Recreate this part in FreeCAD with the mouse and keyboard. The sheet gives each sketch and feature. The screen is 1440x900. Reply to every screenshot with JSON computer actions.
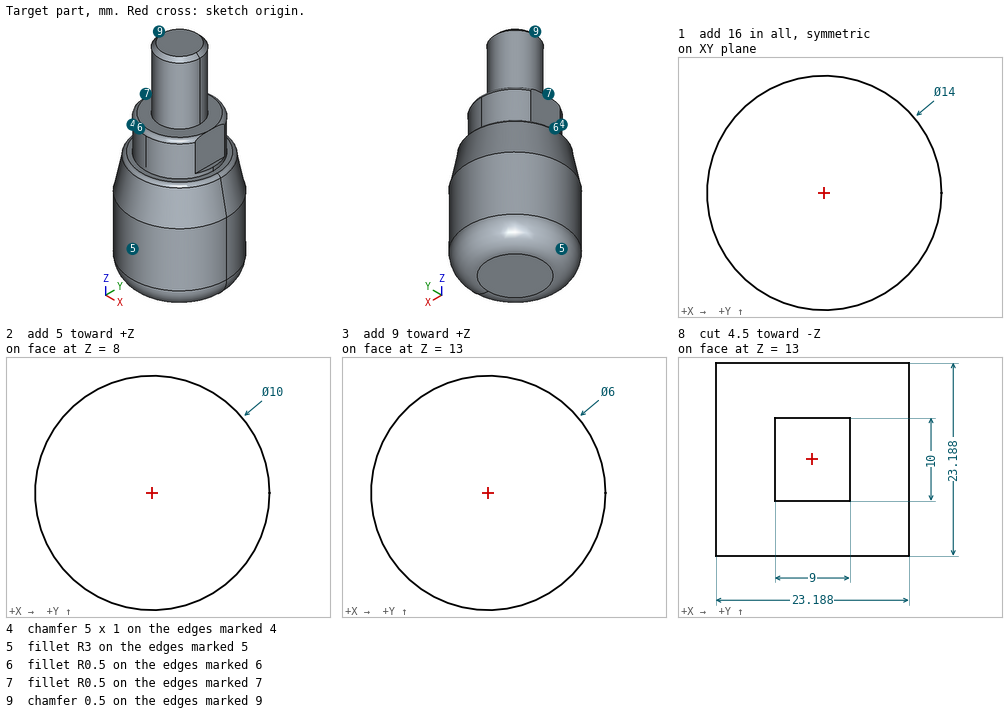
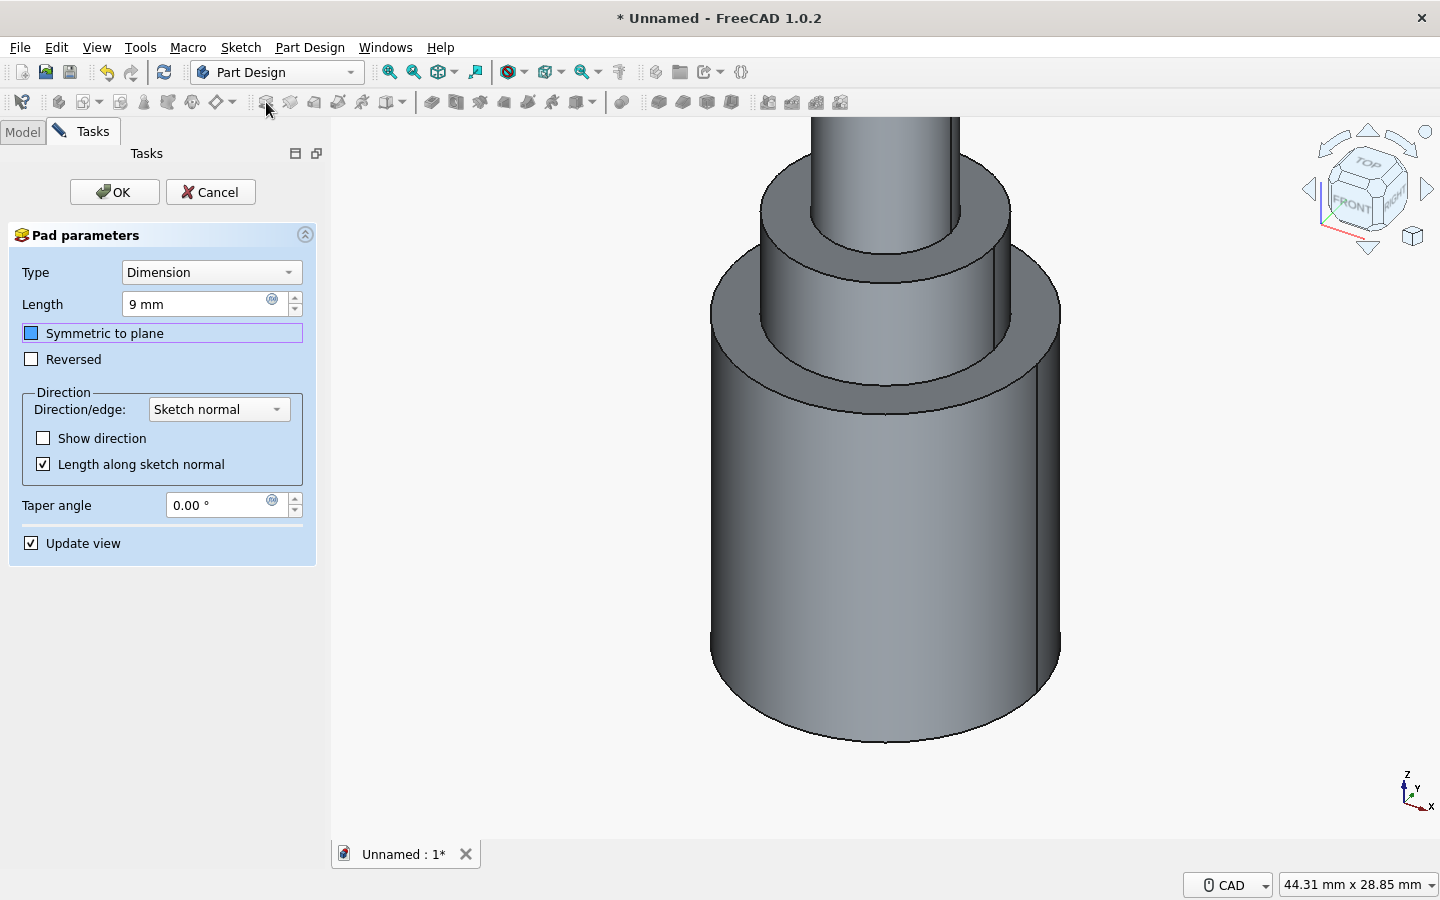
{"action": "left_click", "coordinate": [115, 192]}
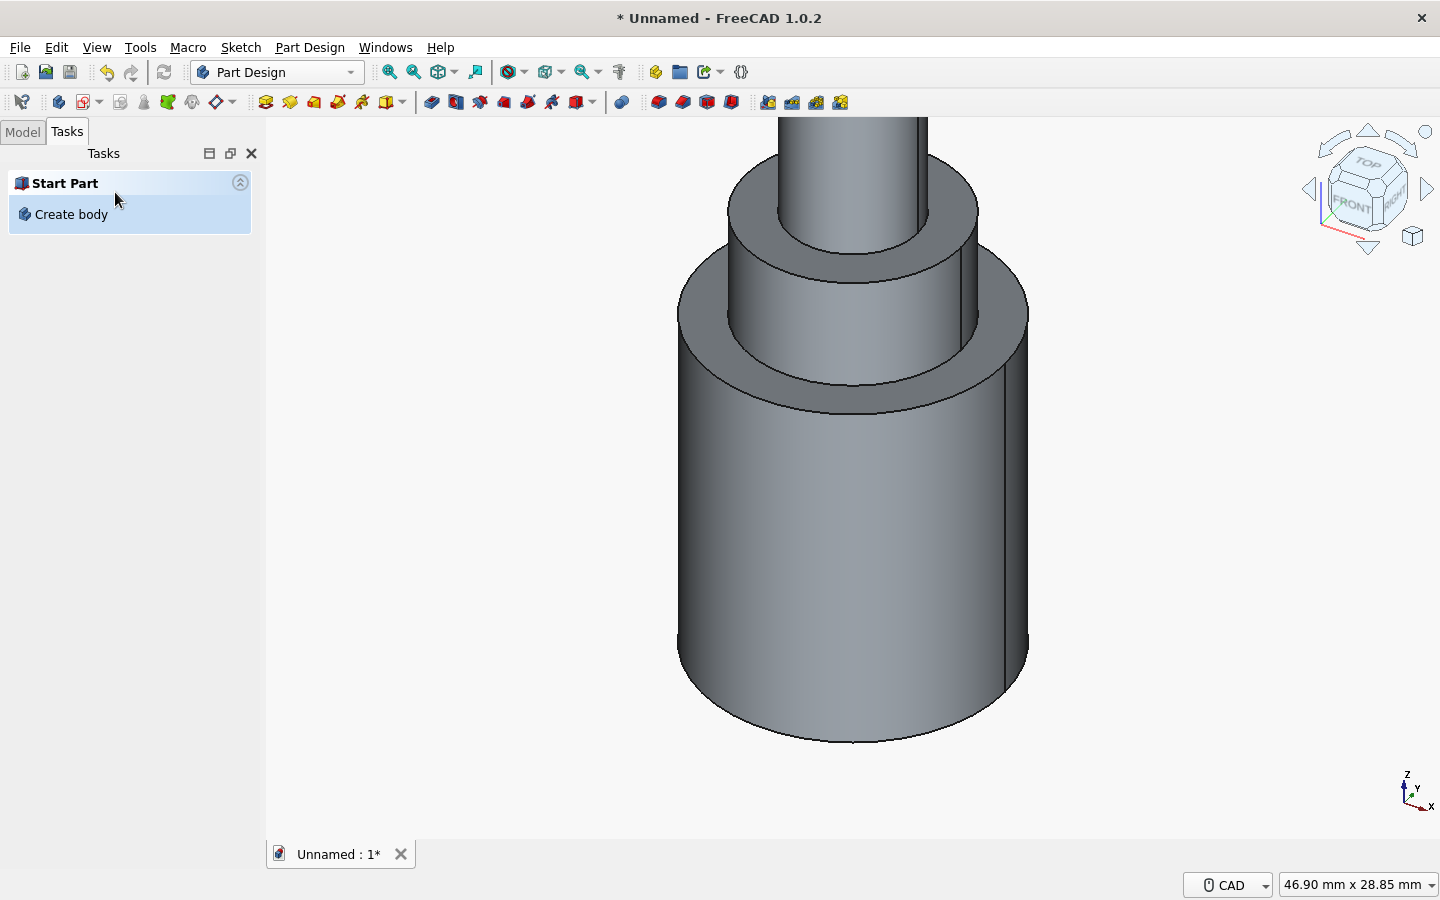
{"action": "key", "text": "v f"}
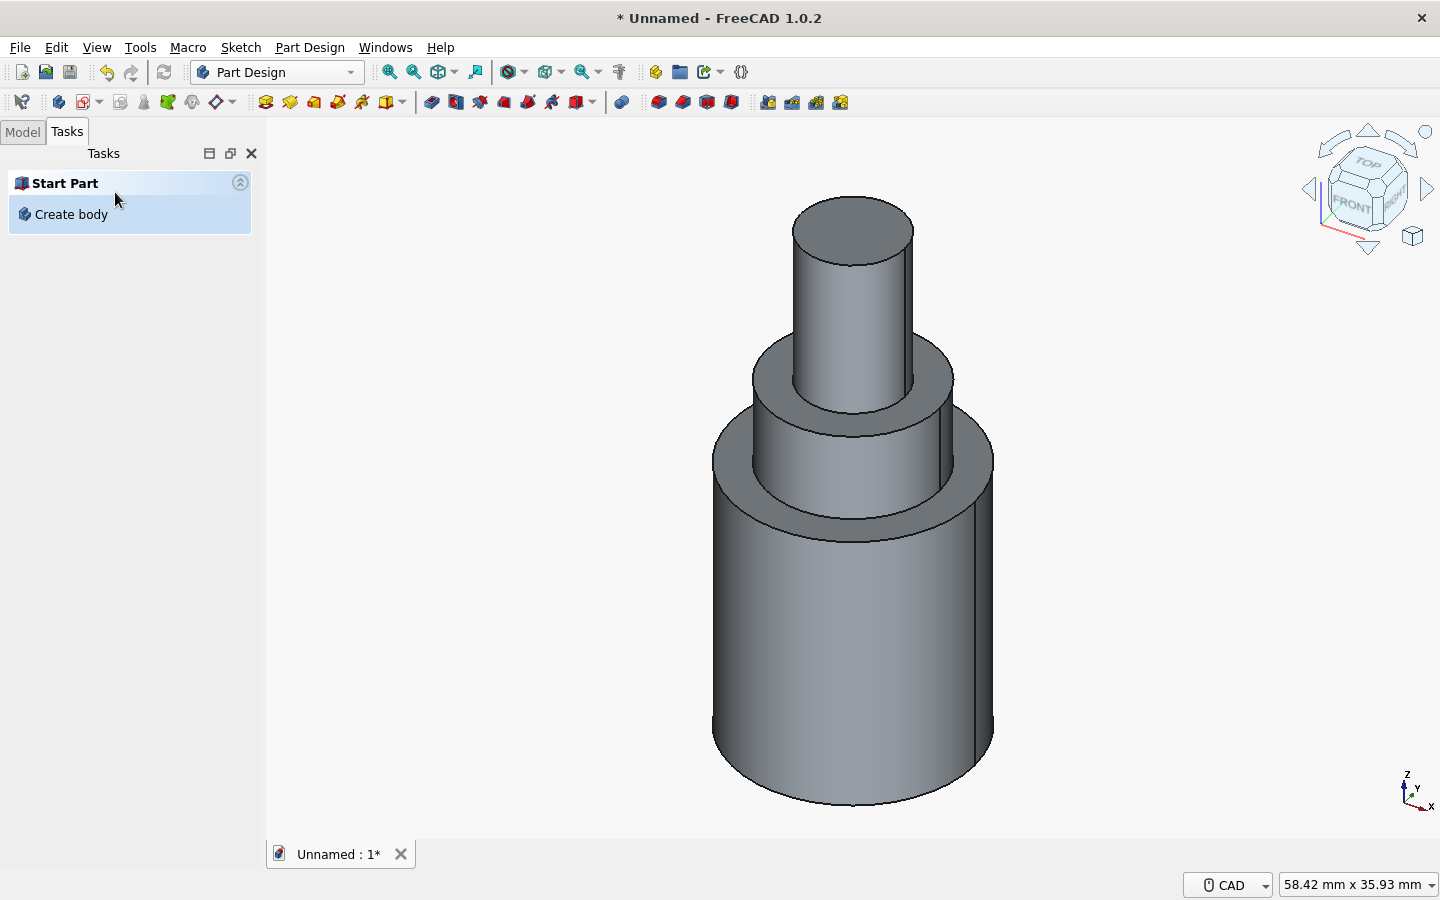
{"action": "left_click", "coordinate": [713, 469]}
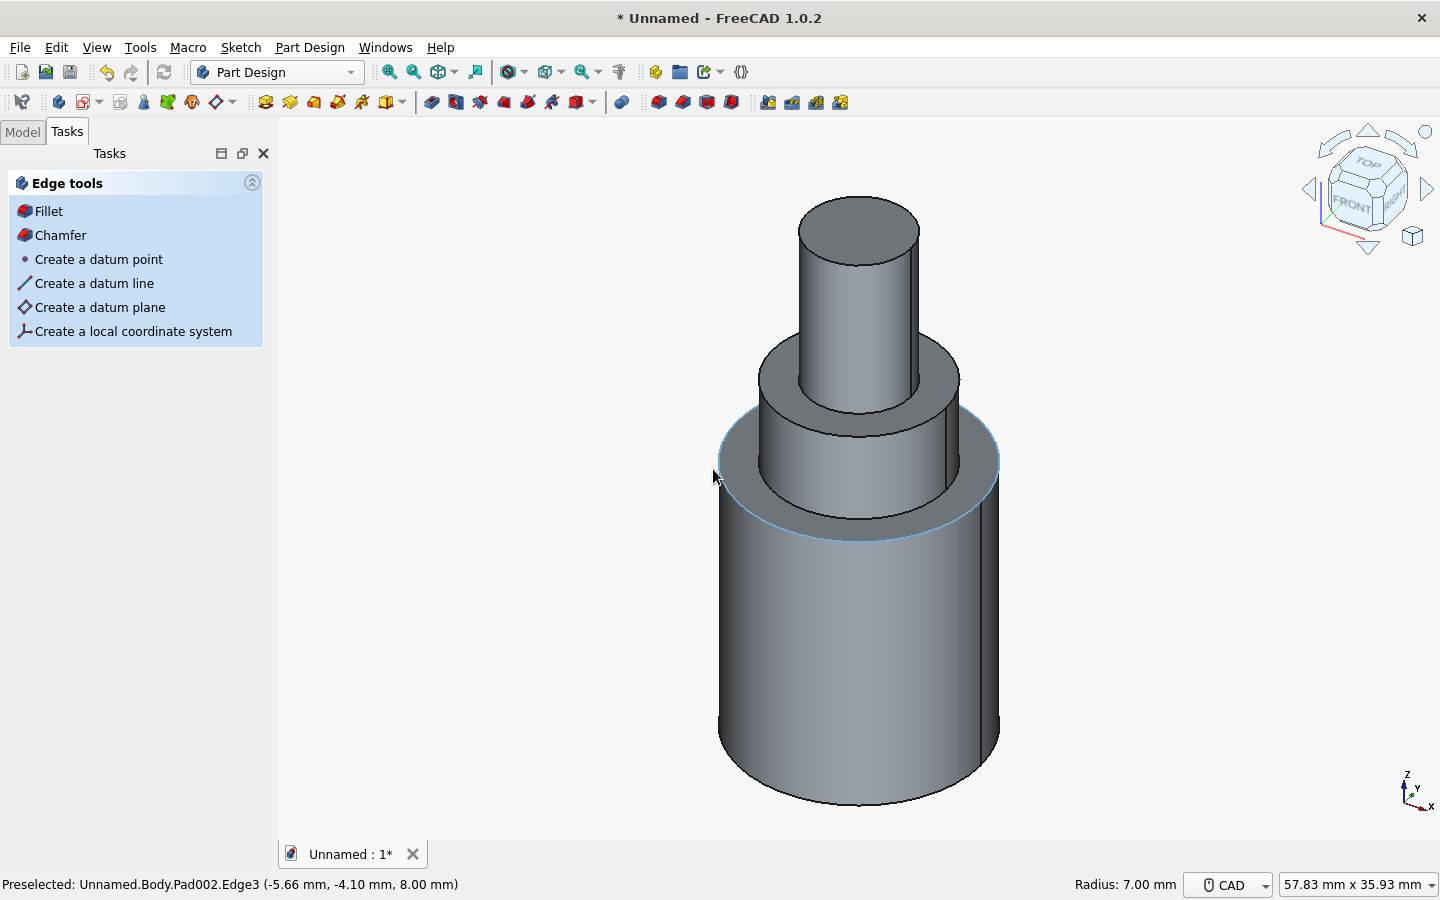
{"action": "left_click", "coordinate": [684, 102]}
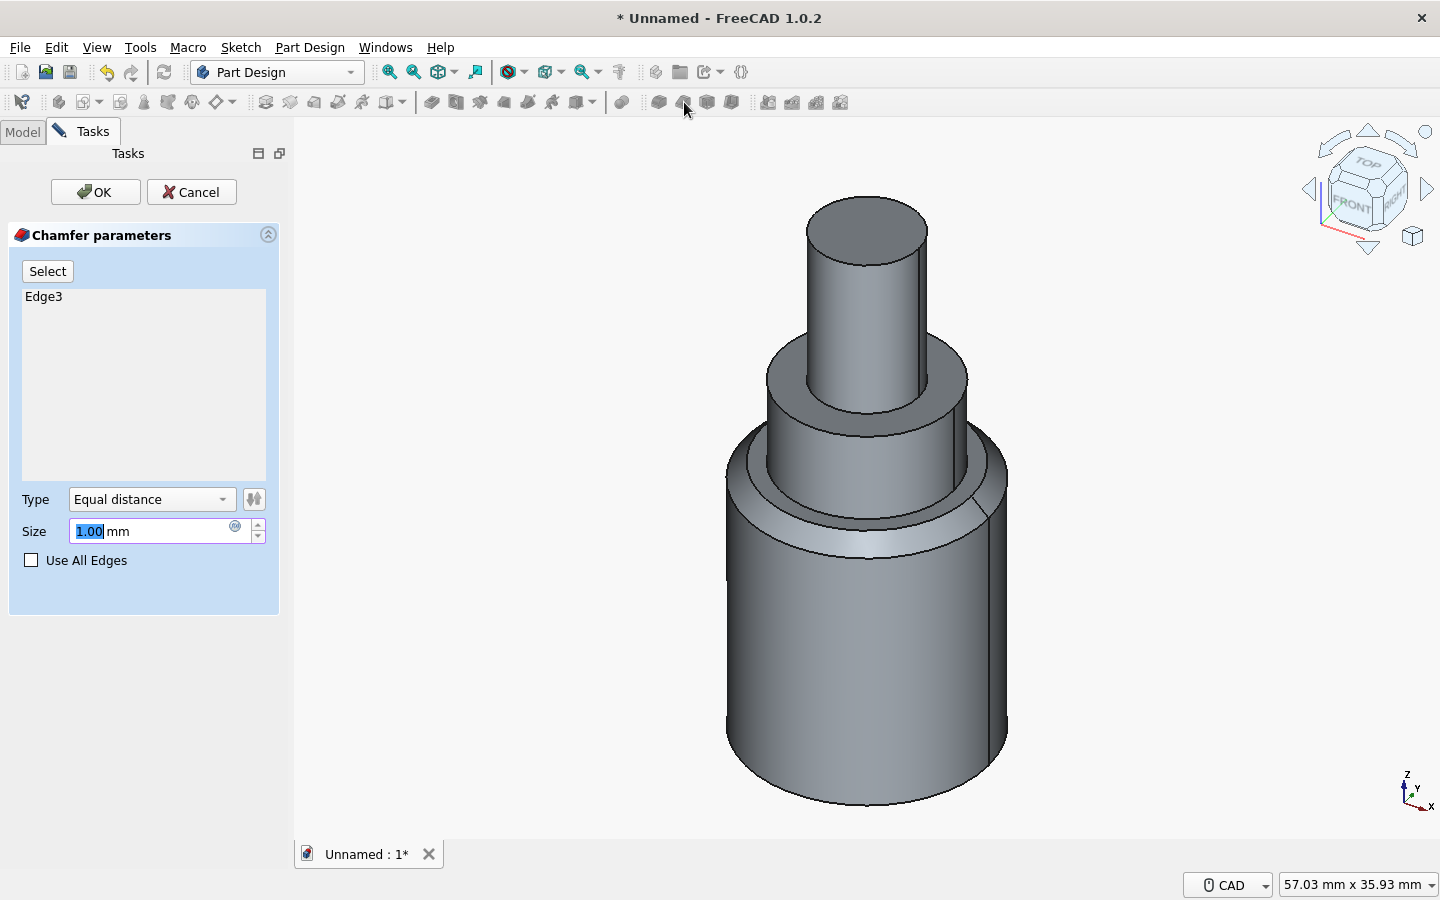
{"action": "type", "text": "5"}
{"action": "key", "text": "Tab"}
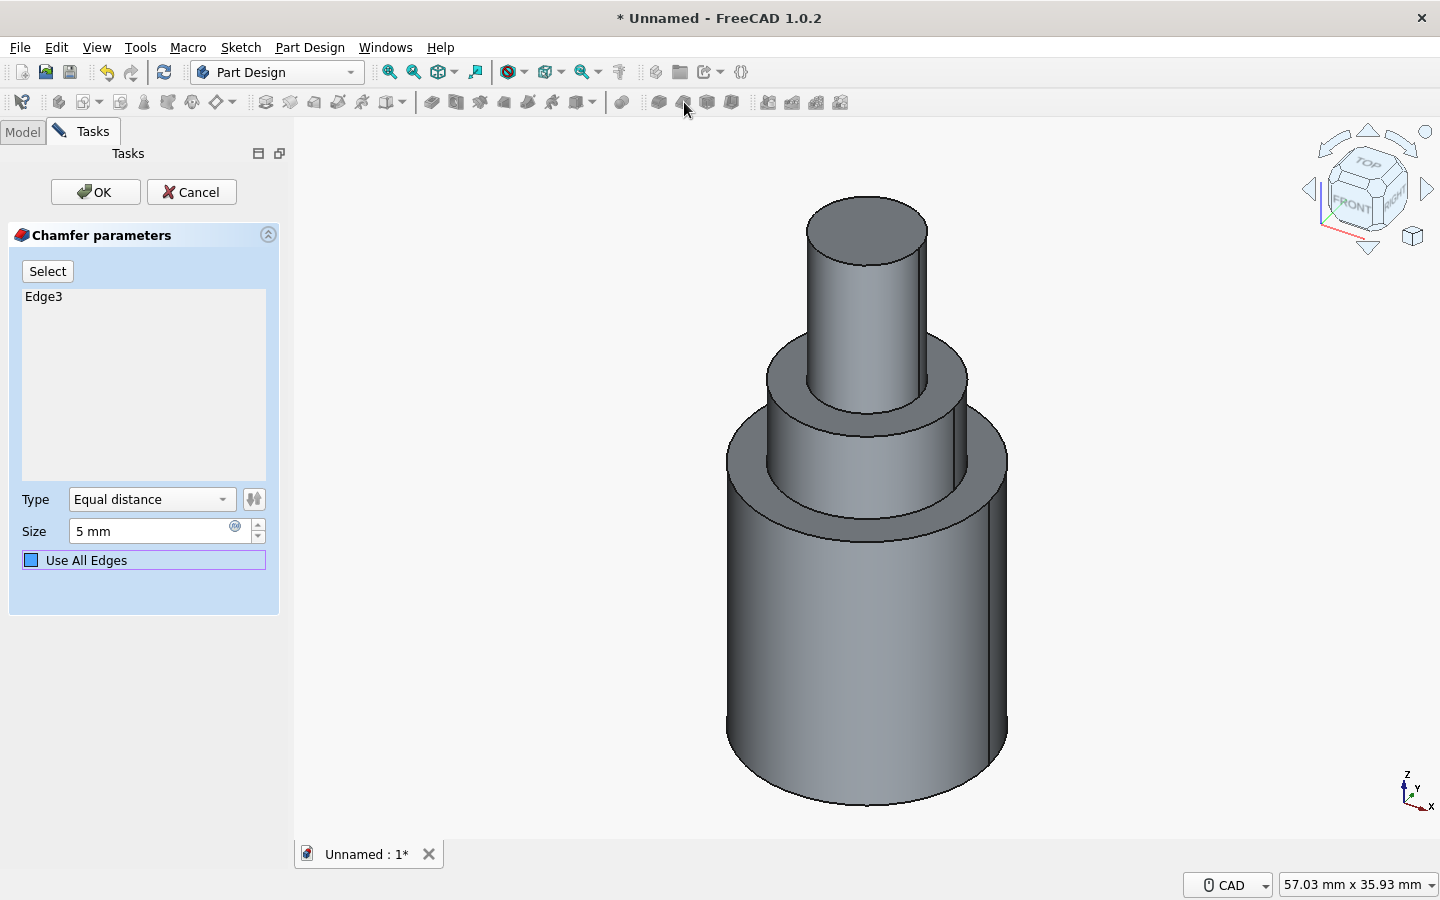
{"action": "left_click", "coordinate": [153, 500]}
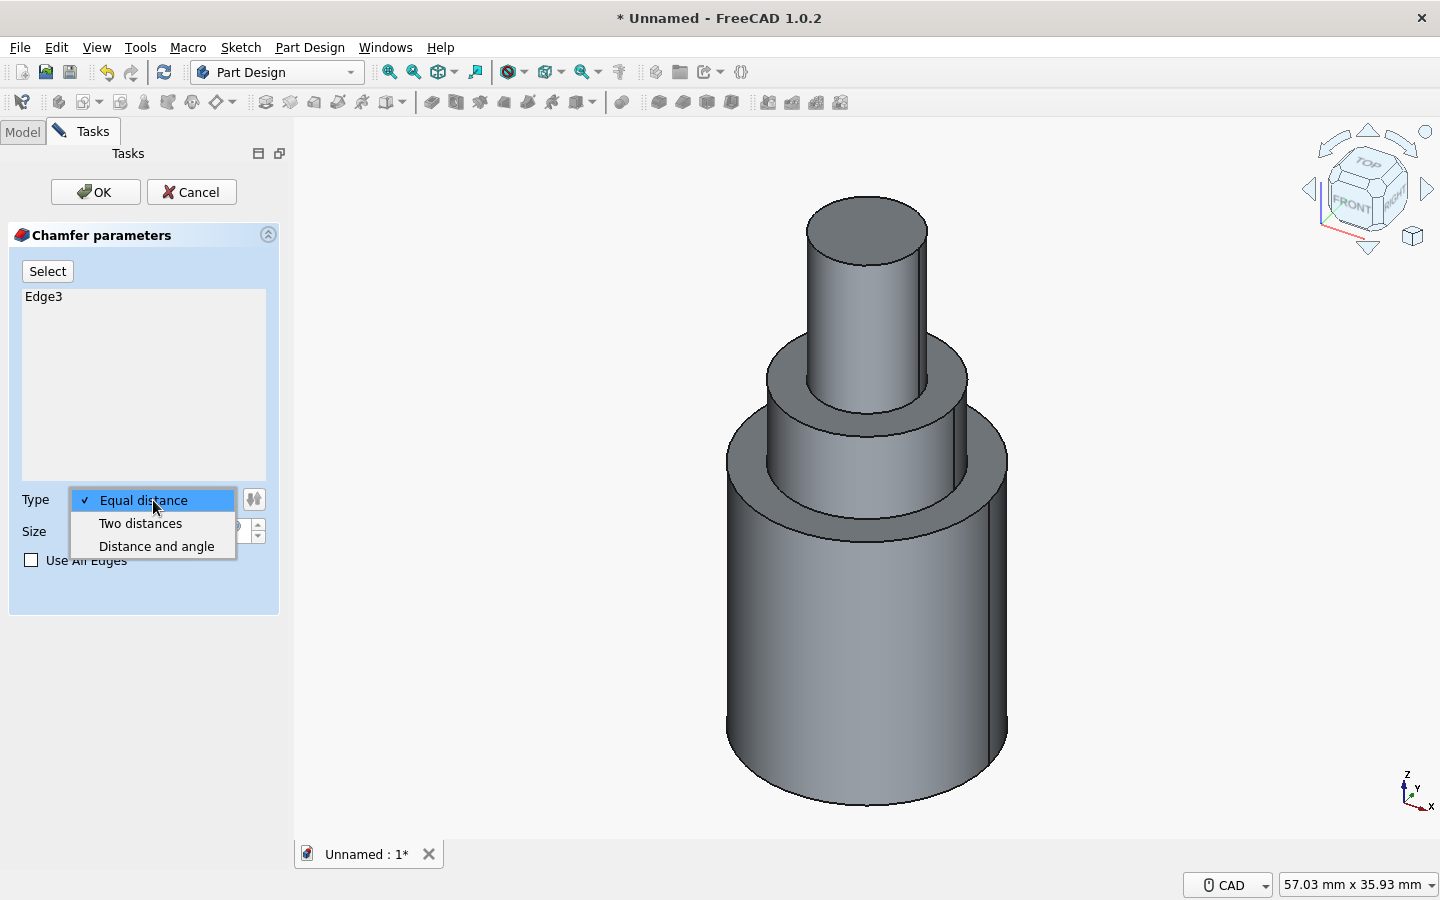
{"action": "left_click", "coordinate": [152, 524]}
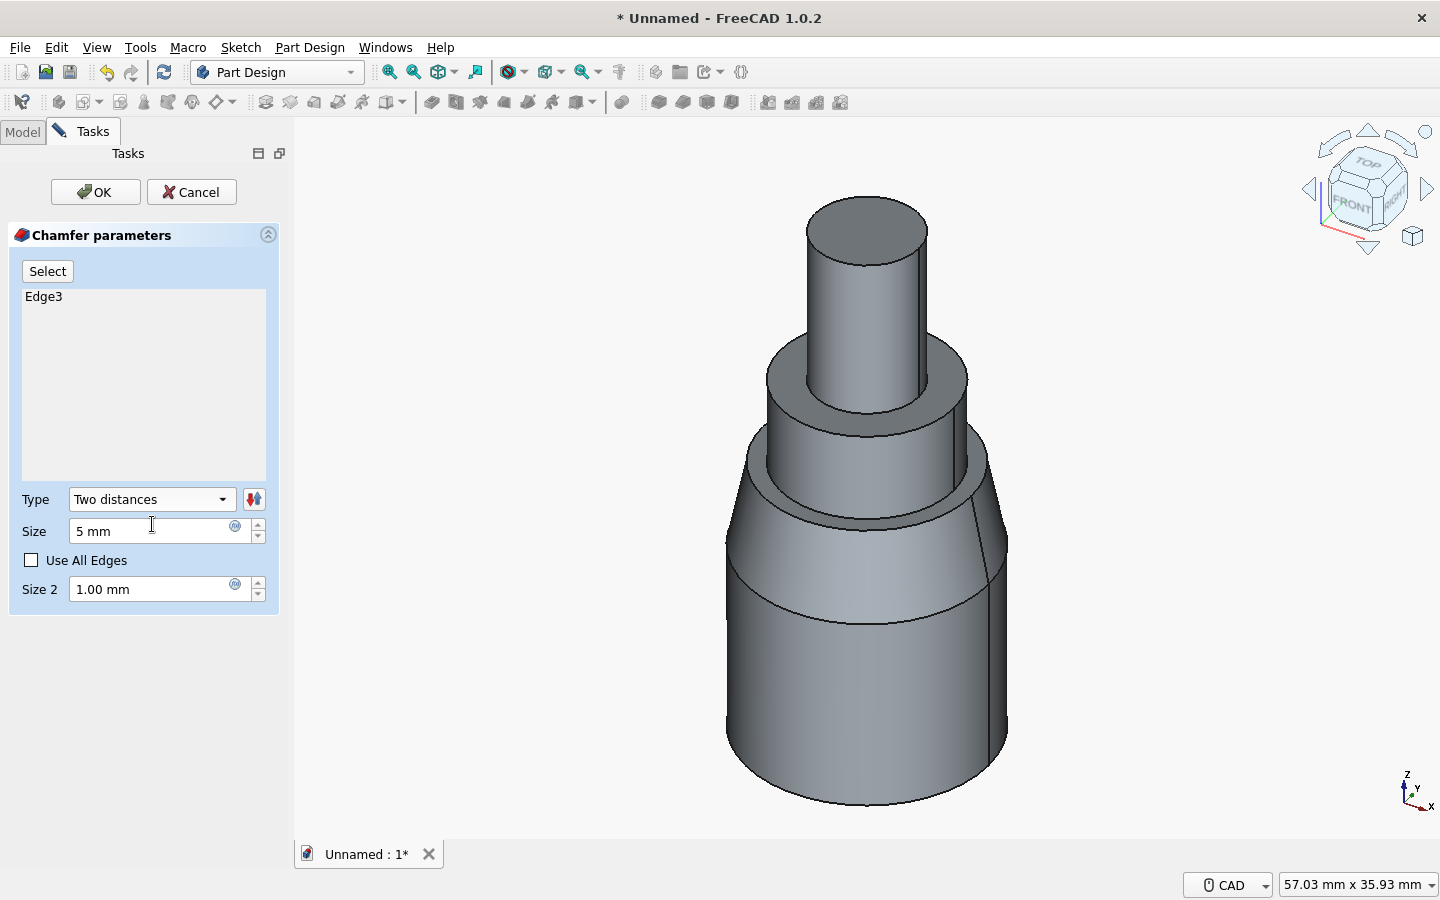
{"action": "triple_click", "coordinate": [160, 589]}